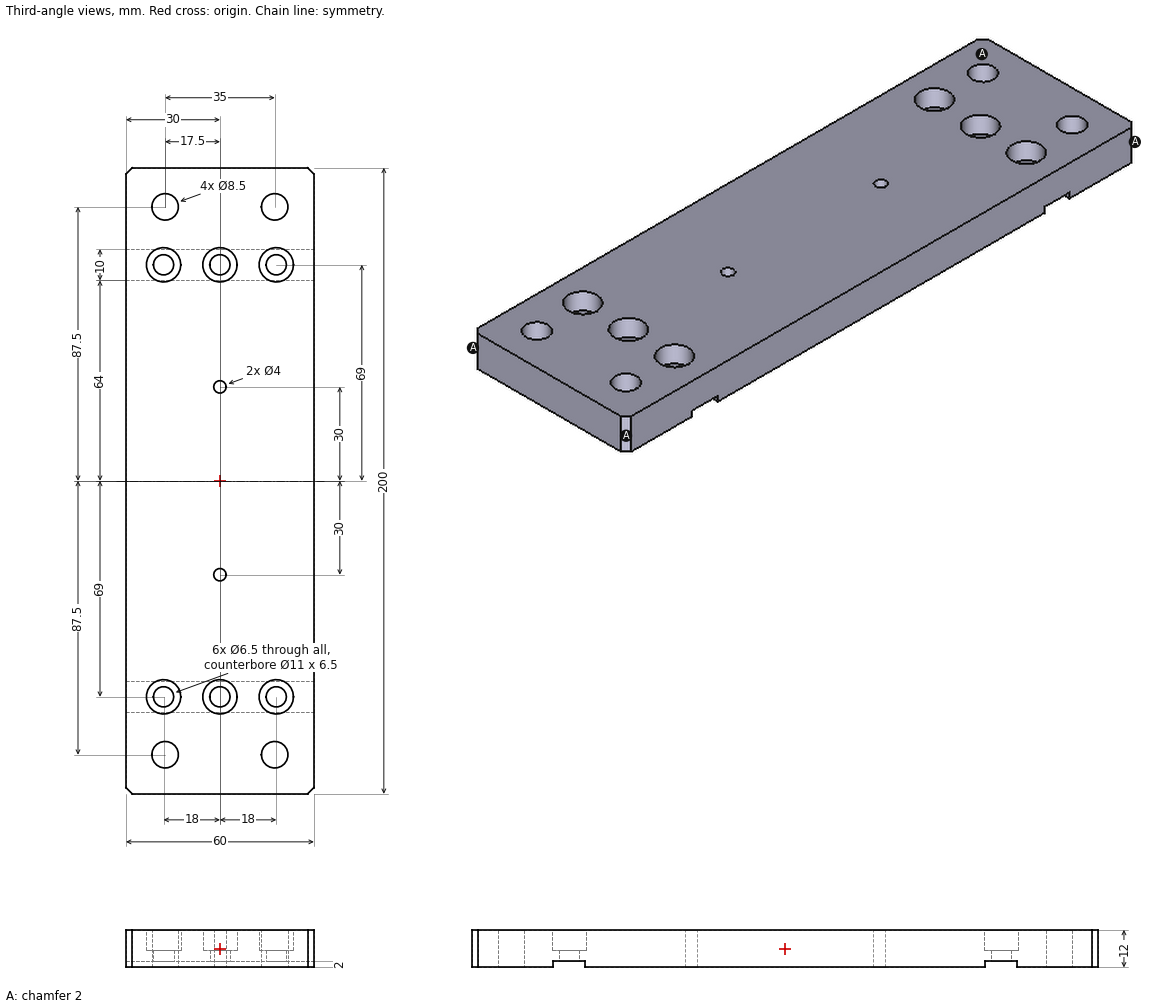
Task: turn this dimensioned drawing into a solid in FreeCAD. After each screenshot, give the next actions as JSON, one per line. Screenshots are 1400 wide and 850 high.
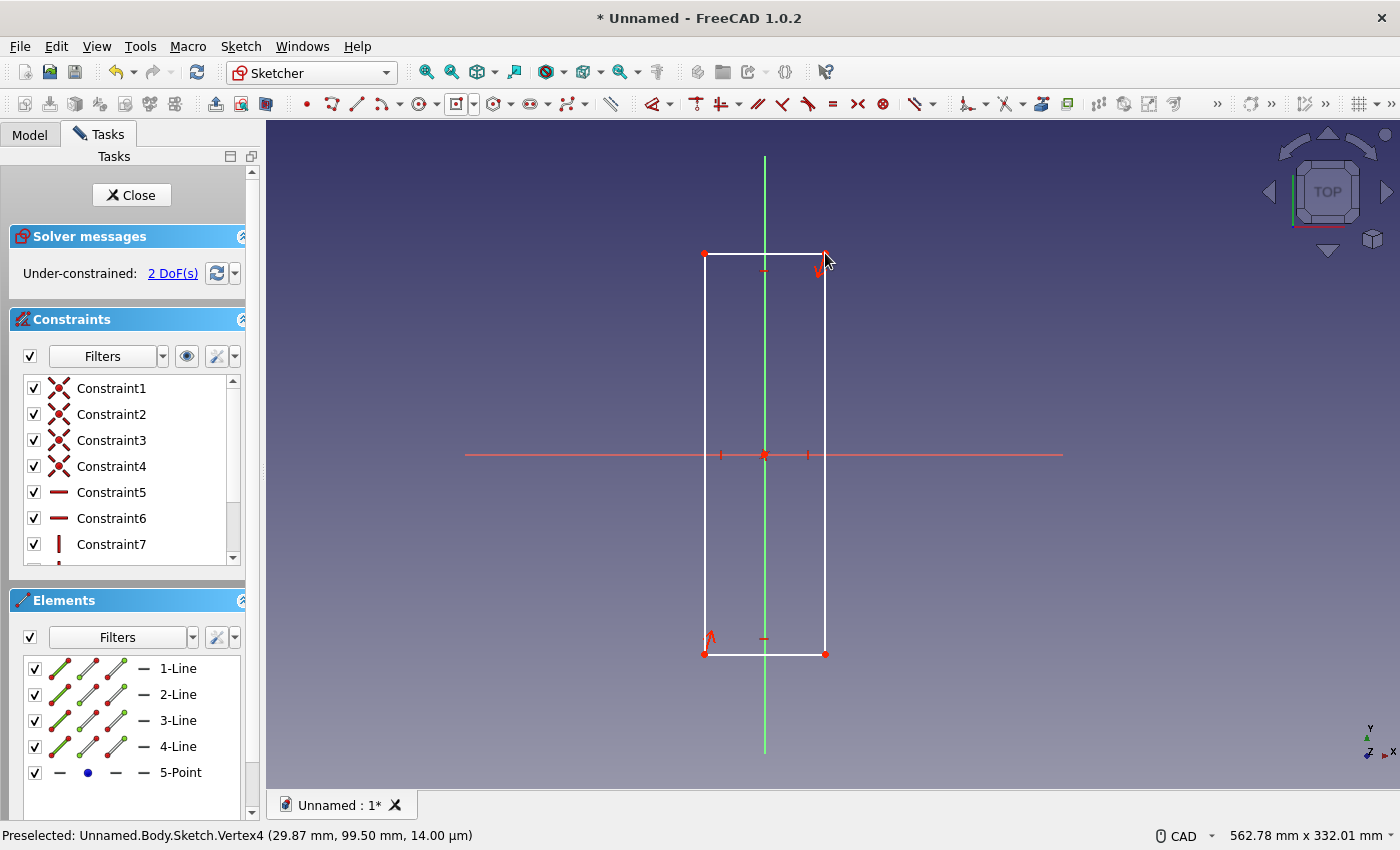
{"action": "left_click", "coordinate": [652, 104]}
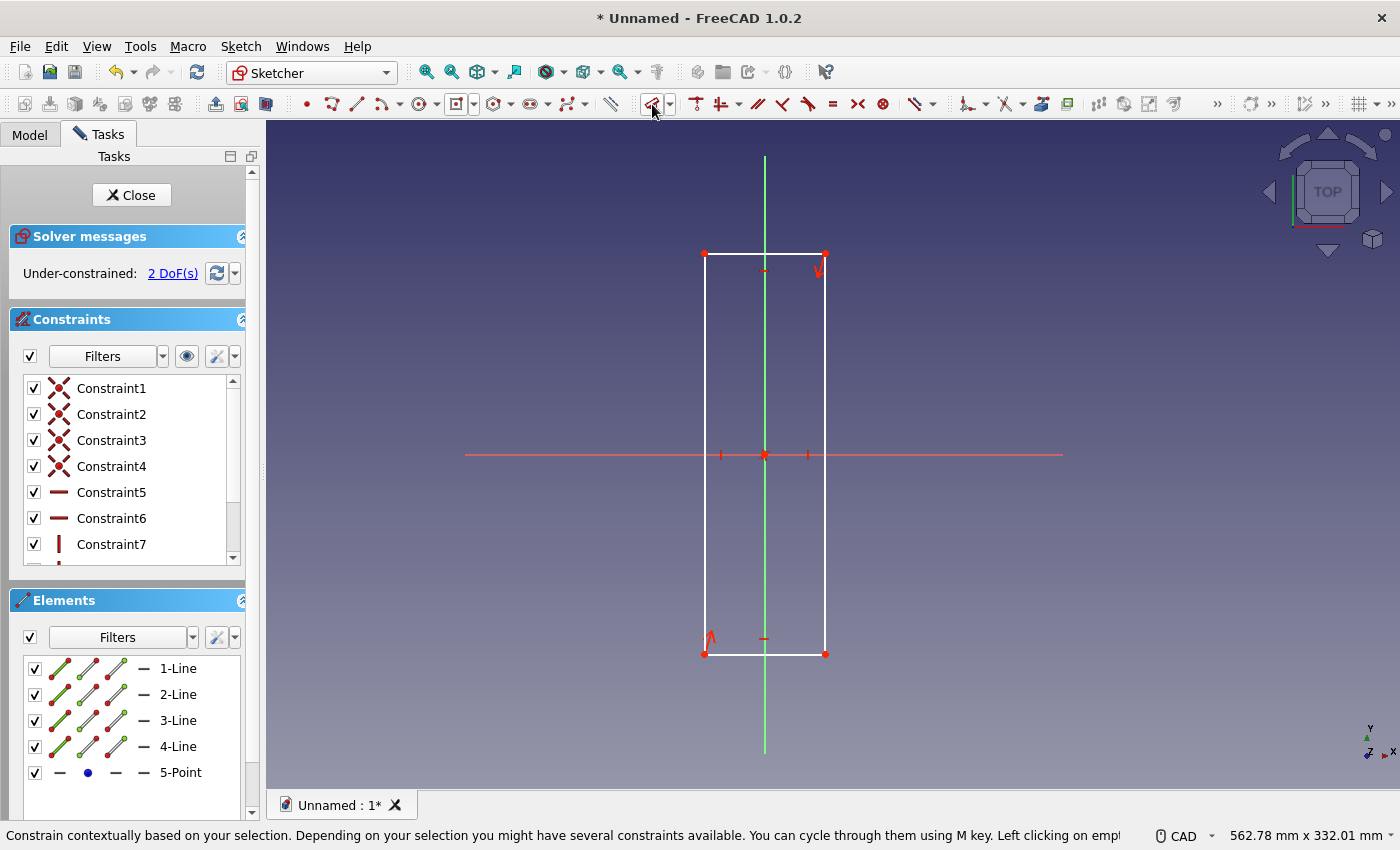
{"action": "left_click", "coordinate": [741, 655]}
{"action": "left_click", "coordinate": [737, 689]}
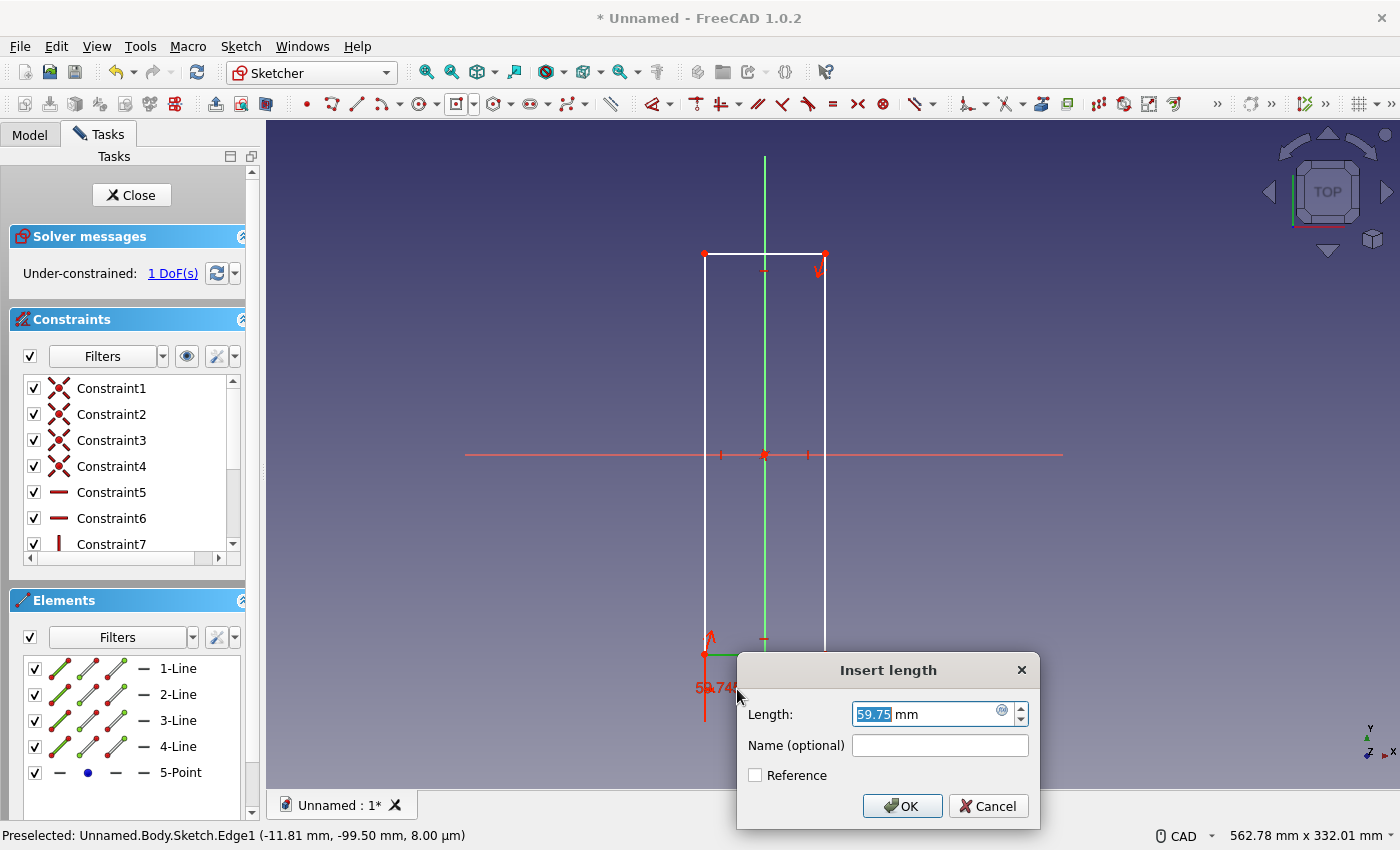
{"action": "type", "text": "60"}
{"action": "key", "text": "Return"}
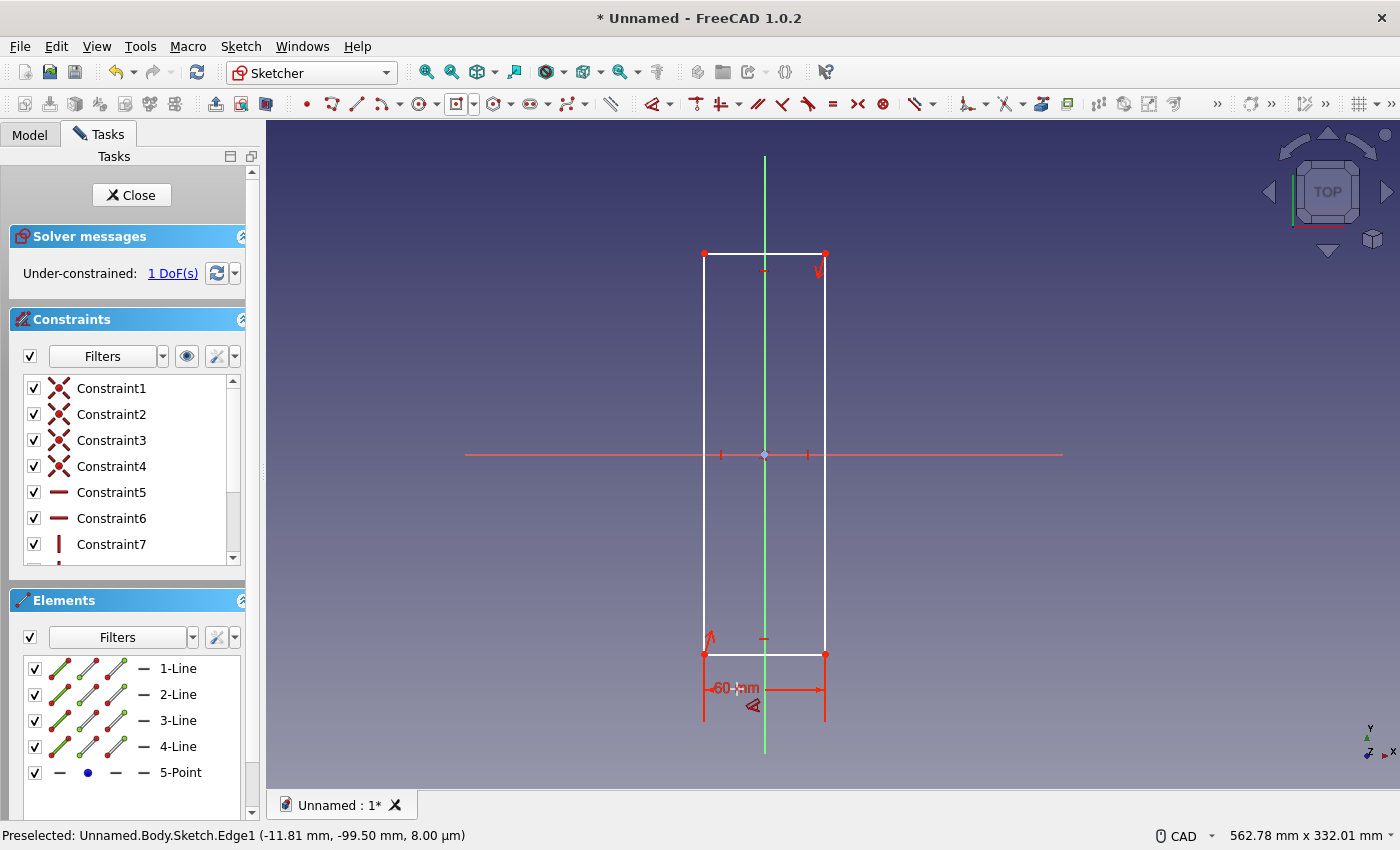
{"action": "left_click", "coordinate": [825, 535]}
{"action": "left_click", "coordinate": [859, 362]}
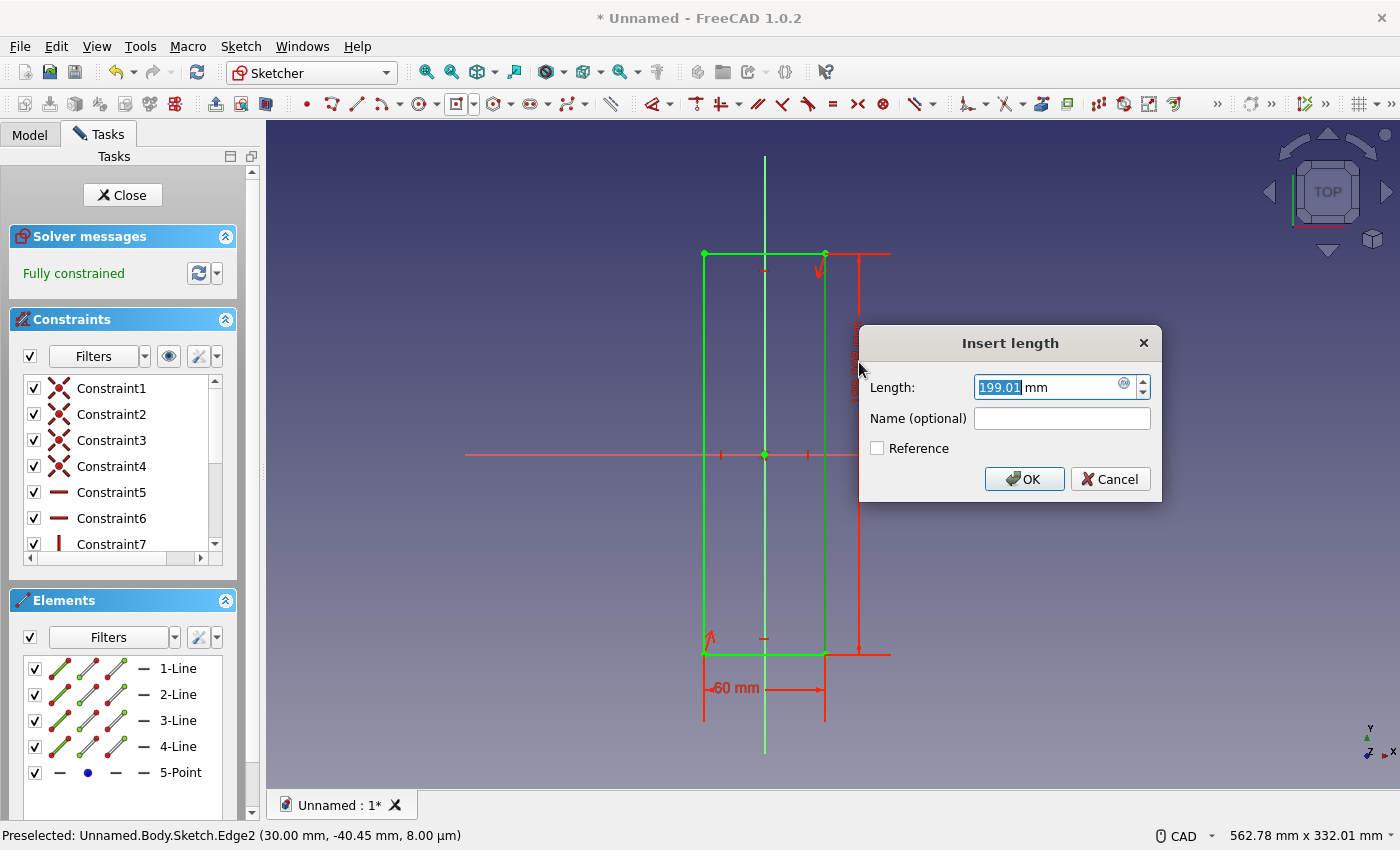
{"action": "type", "text": "200"}
{"action": "key", "text": "Return"}
{"action": "key", "text": "Escape"}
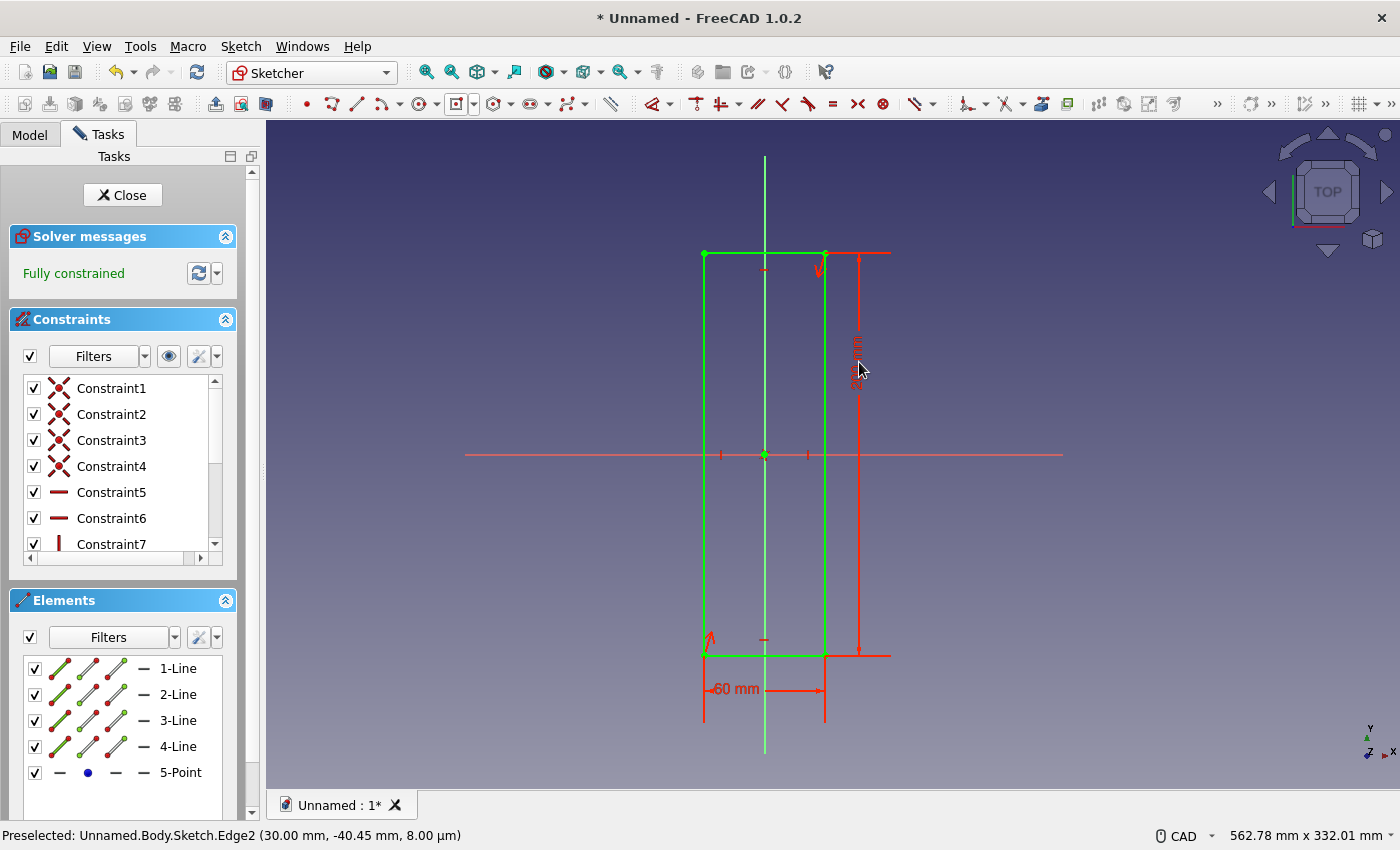
{"action": "left_click", "coordinate": [123, 195]}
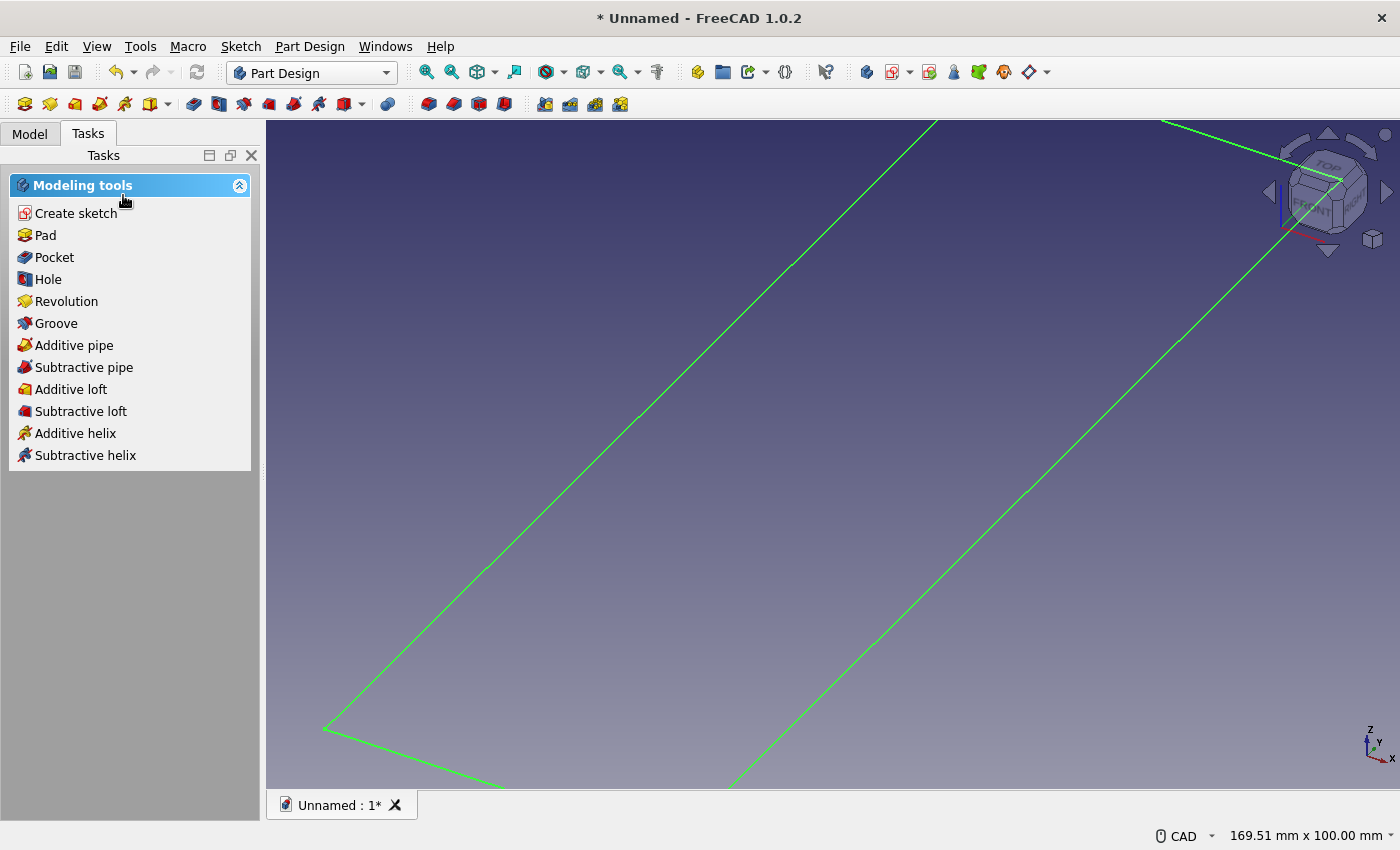
{"action": "left_click", "coordinate": [25, 104]}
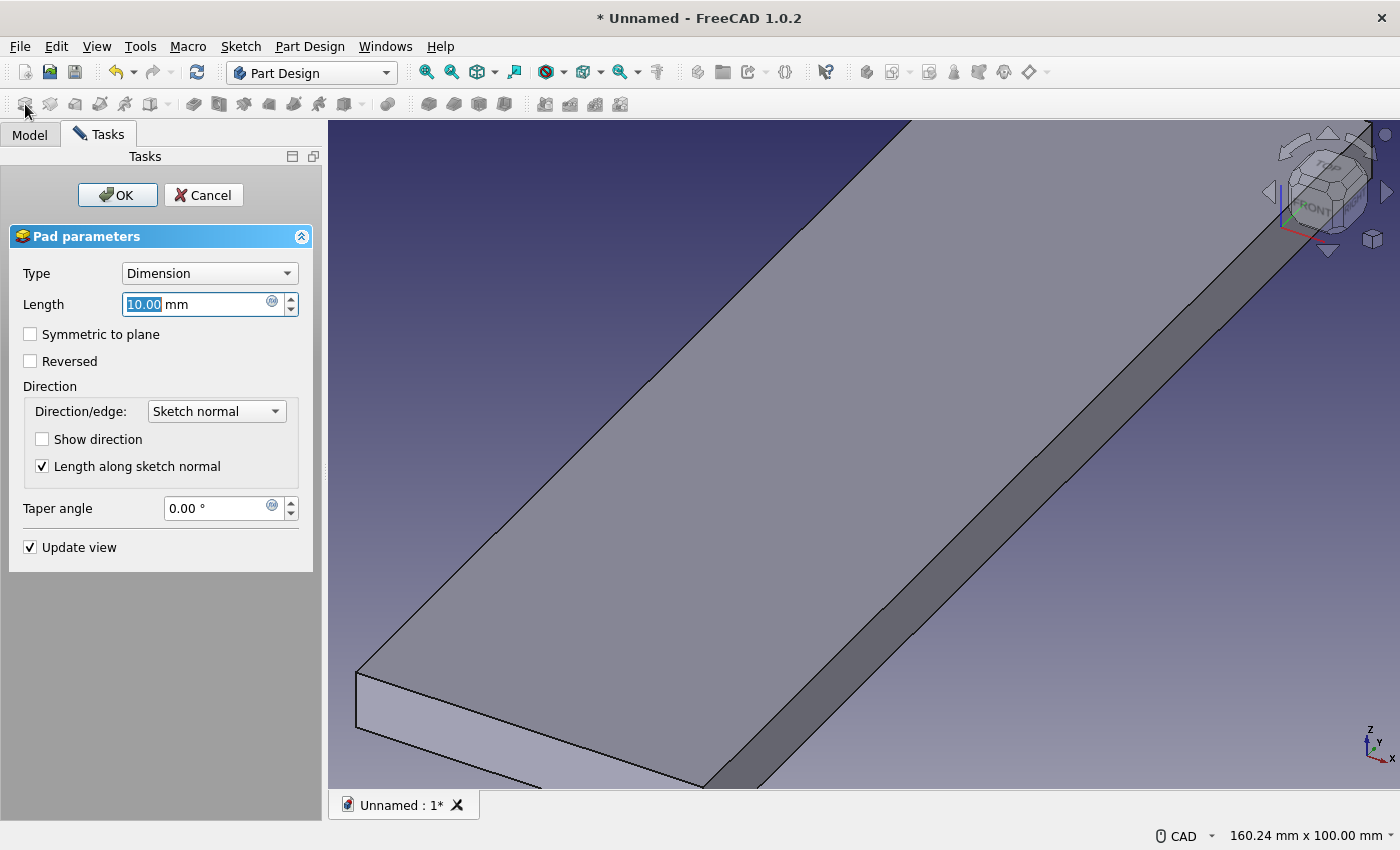
{"action": "type", "text": "12"}
{"action": "key", "text": "Tab"}